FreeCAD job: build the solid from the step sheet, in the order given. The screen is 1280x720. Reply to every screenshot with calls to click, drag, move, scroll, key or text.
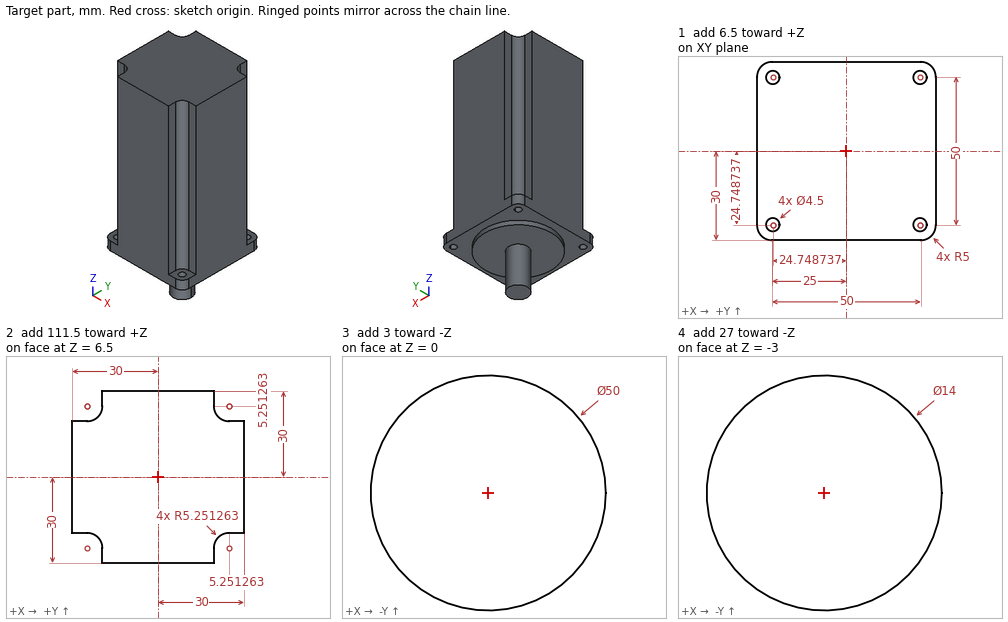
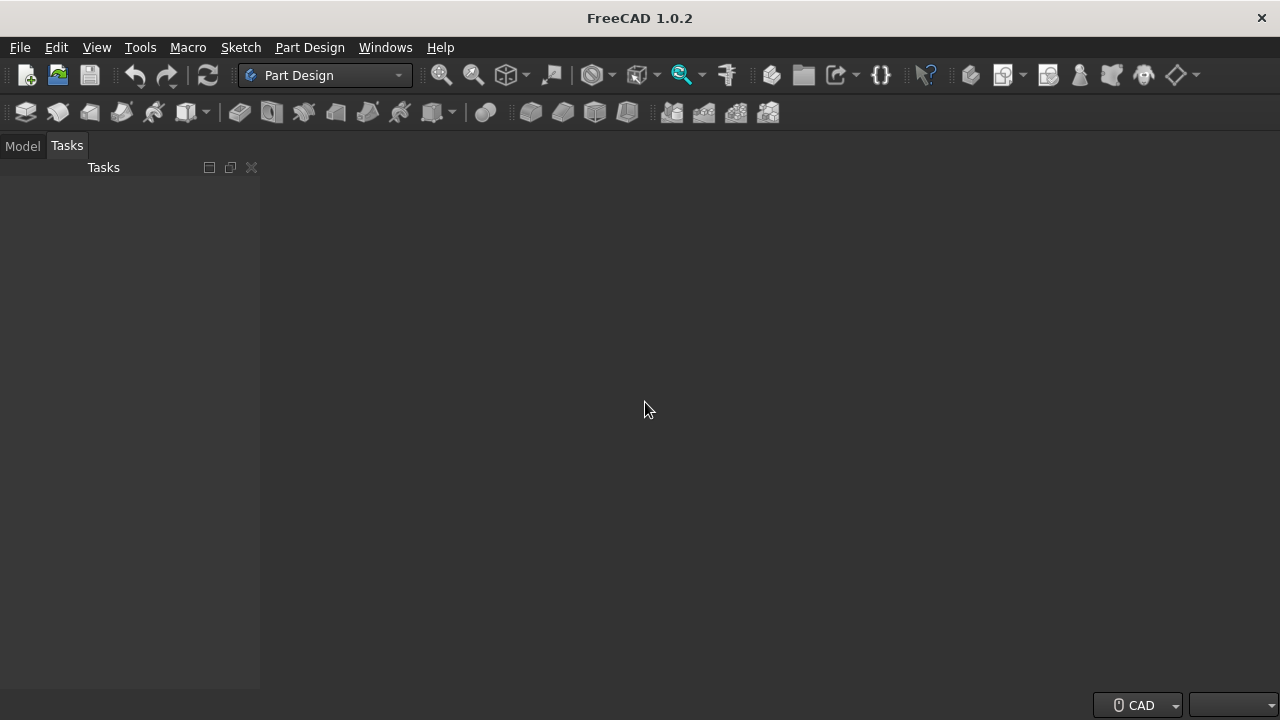
key(ctrl+n)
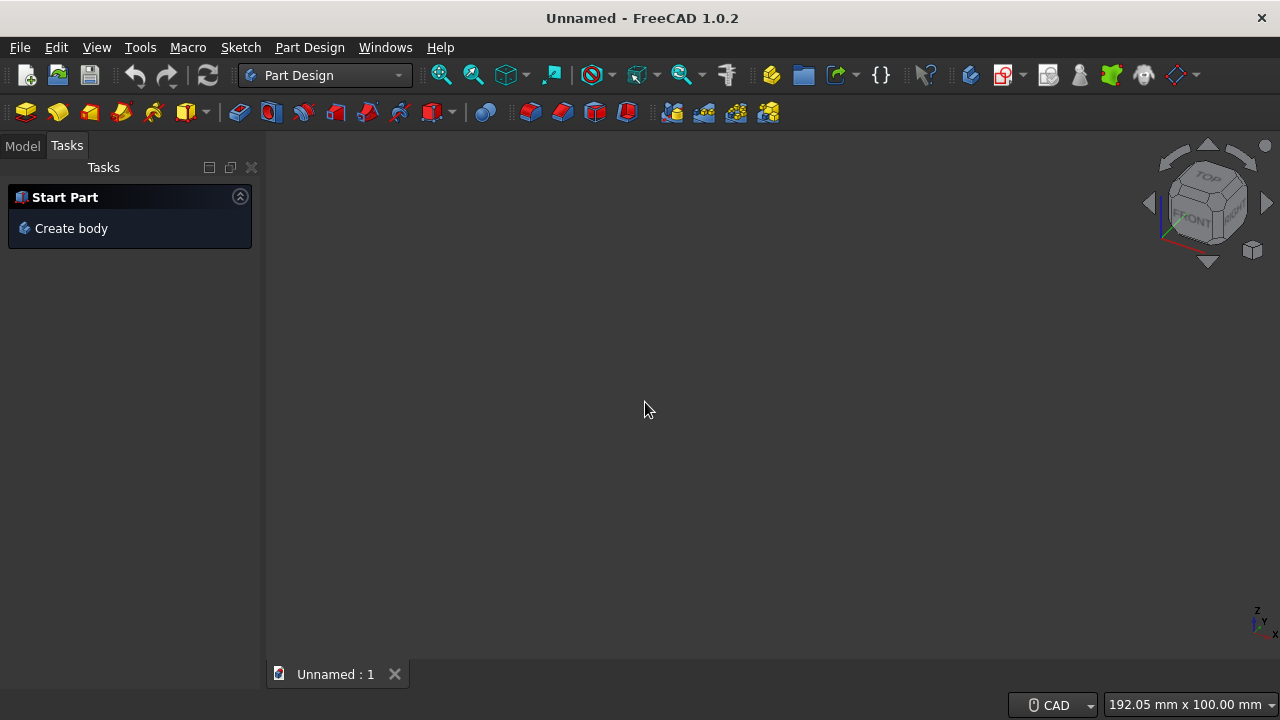
click(1004, 76)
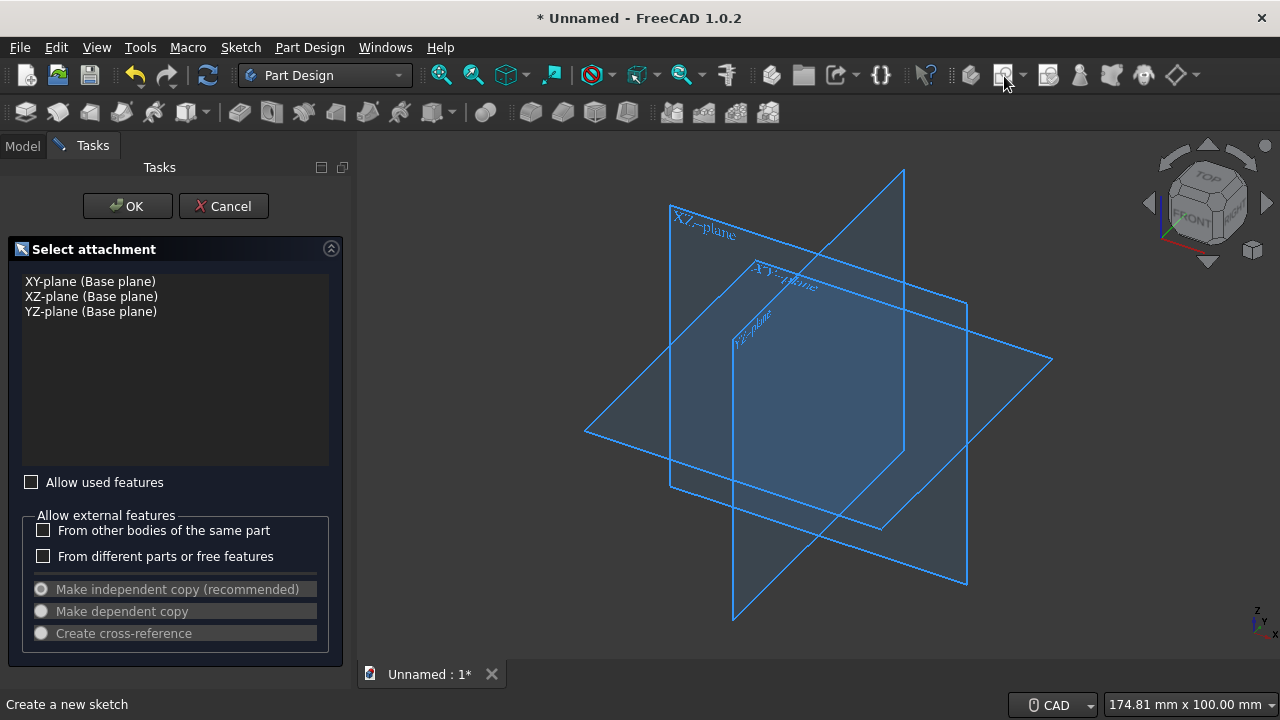
click(82, 282)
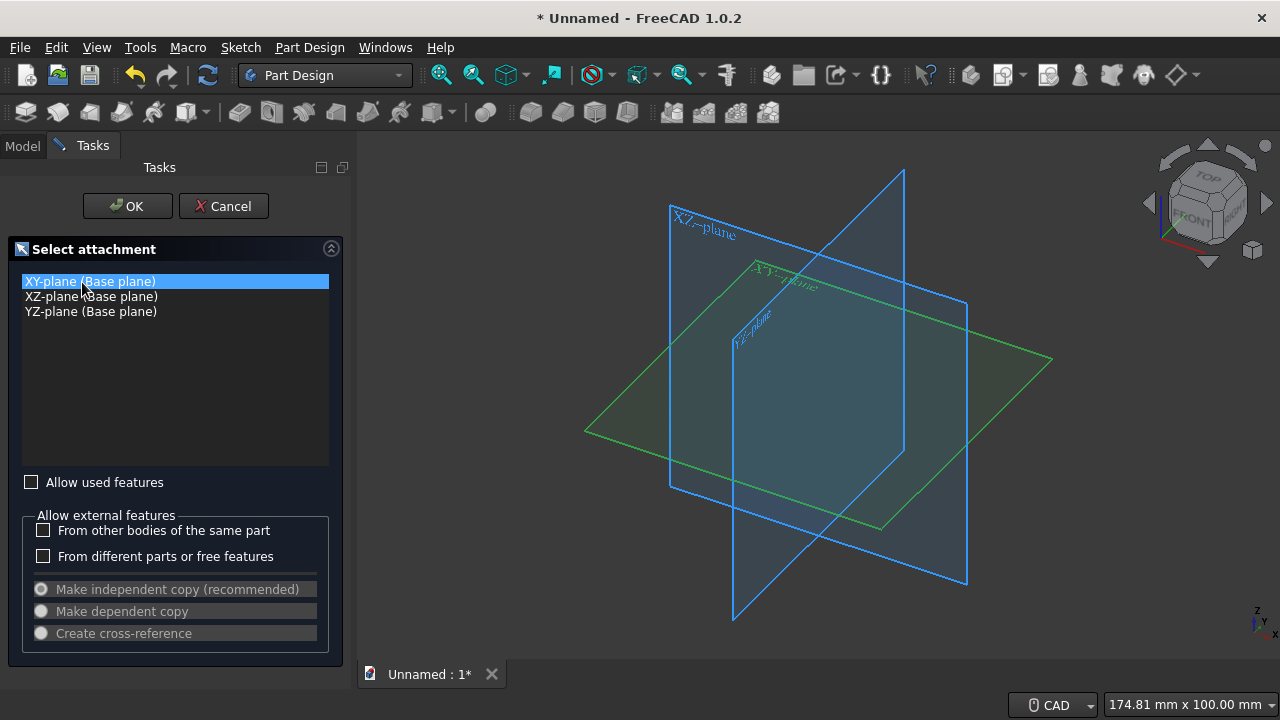
click(128, 206)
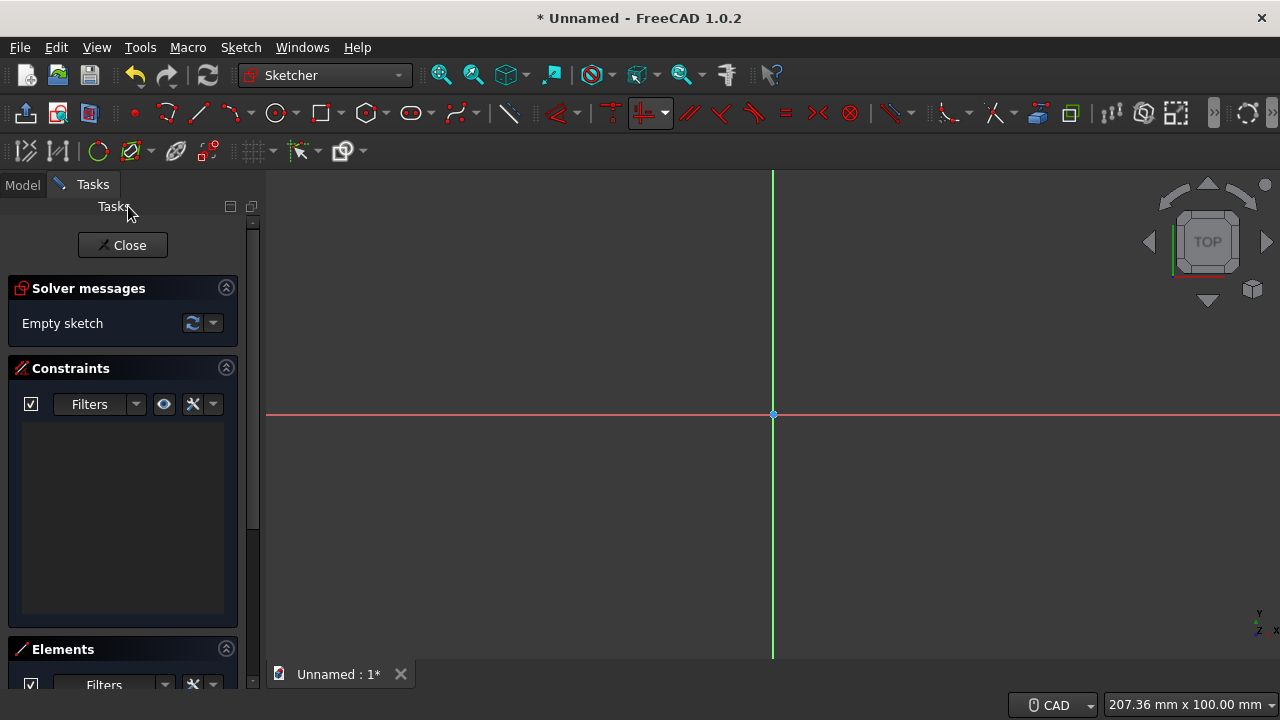
key(g)
key(l)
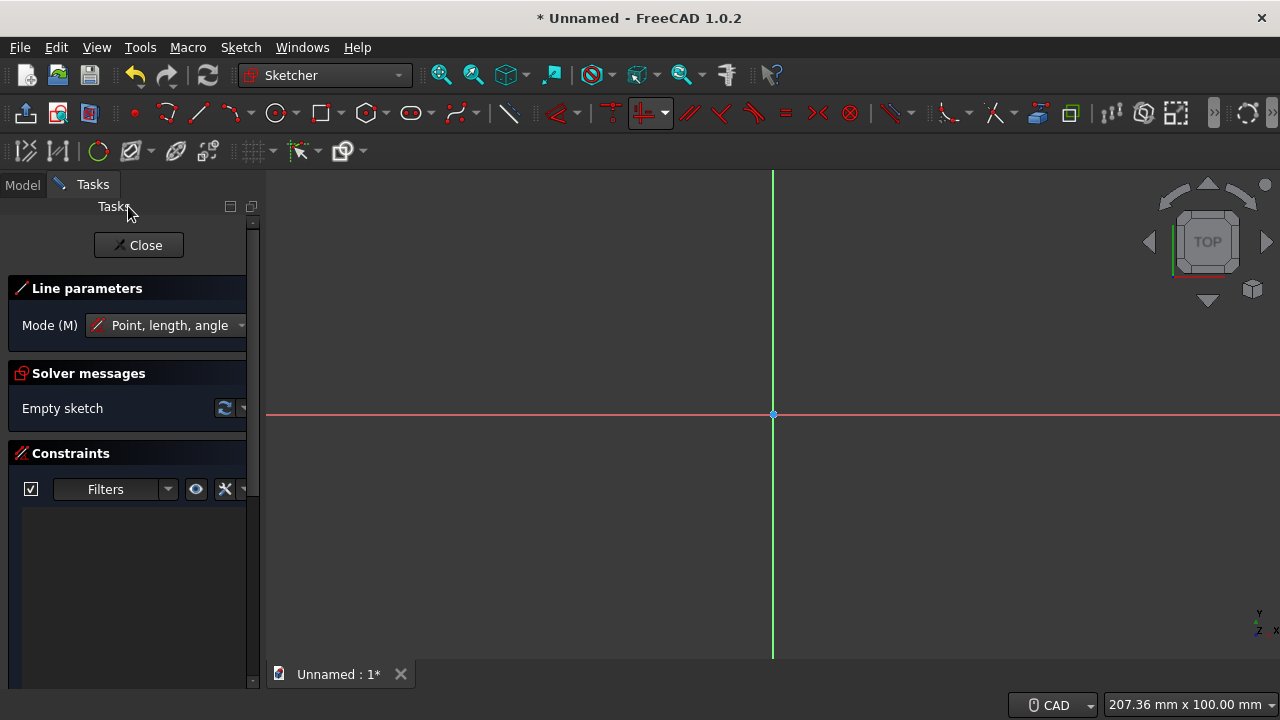
click(651, 561)
click(895, 561)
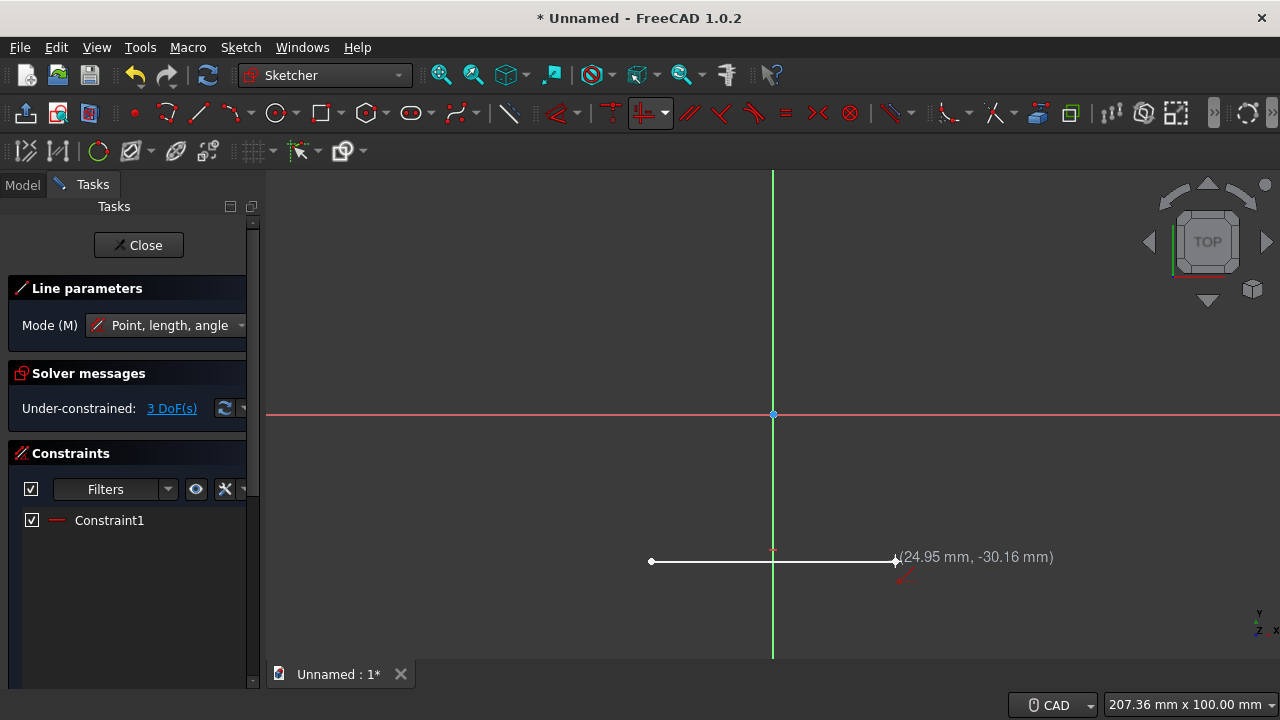
click(920, 537)
click(920, 292)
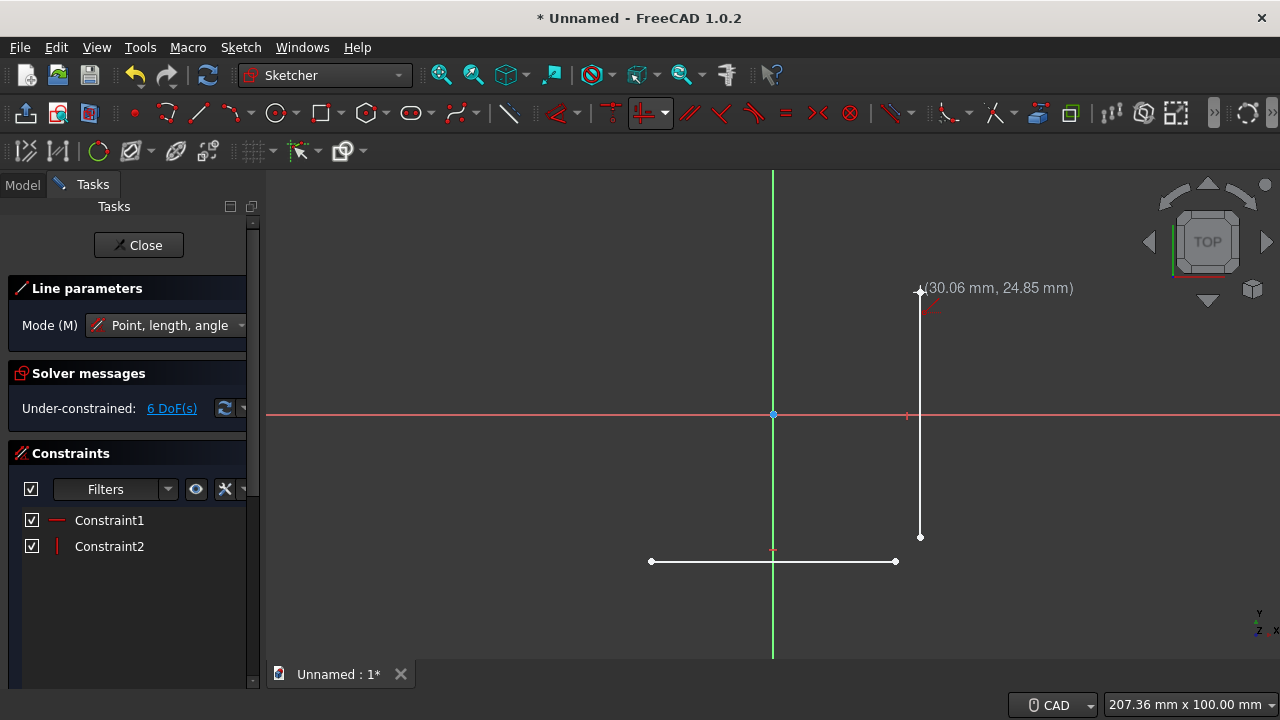
click(895, 268)
click(651, 268)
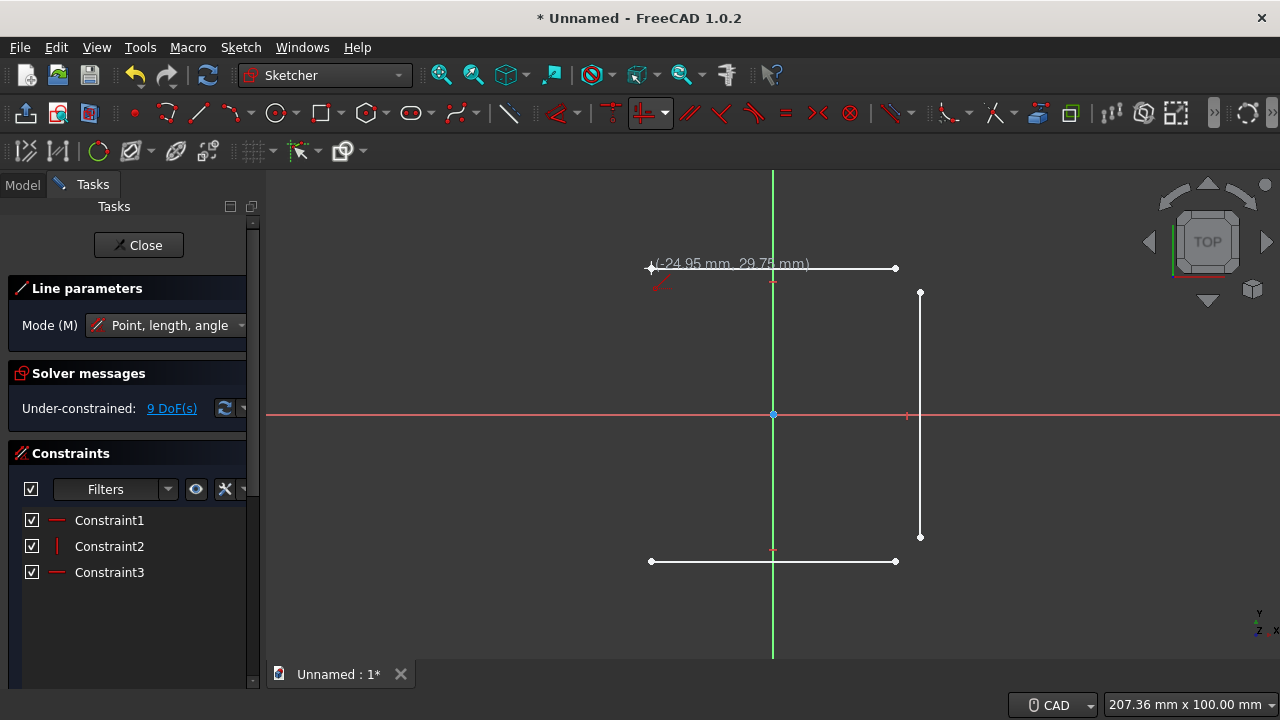
click(626, 292)
click(626, 537)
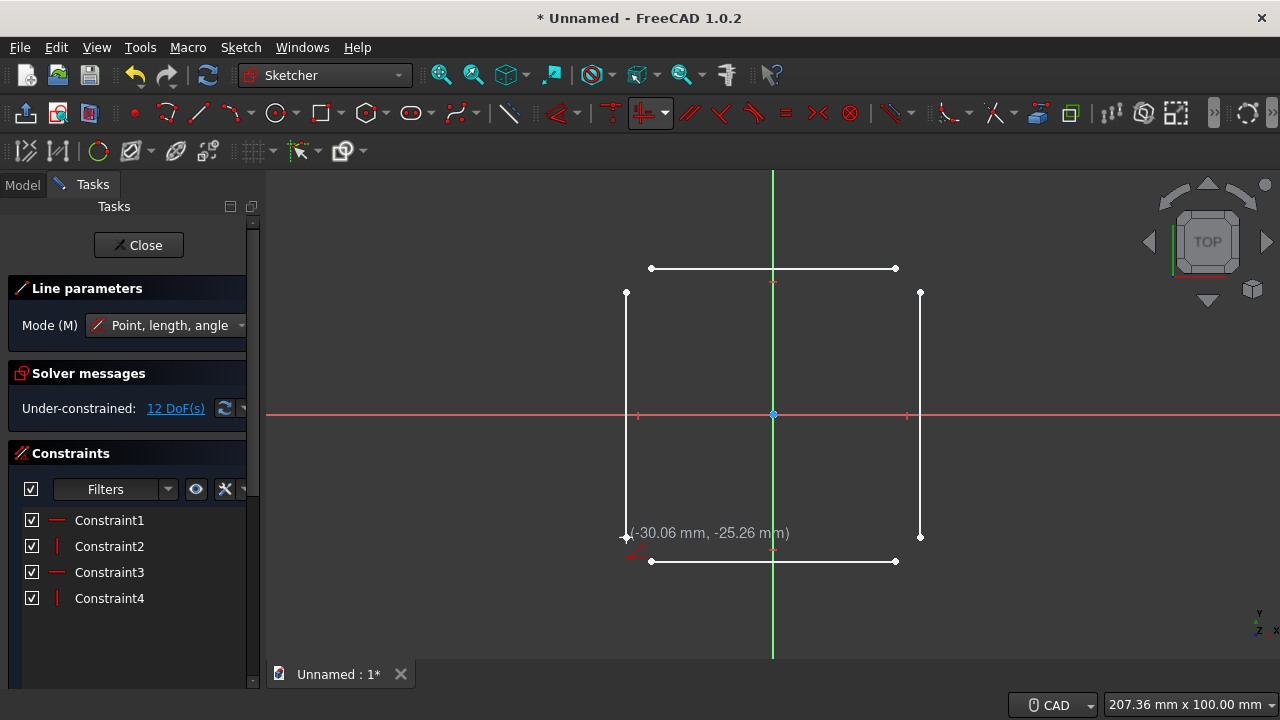
click(232, 114)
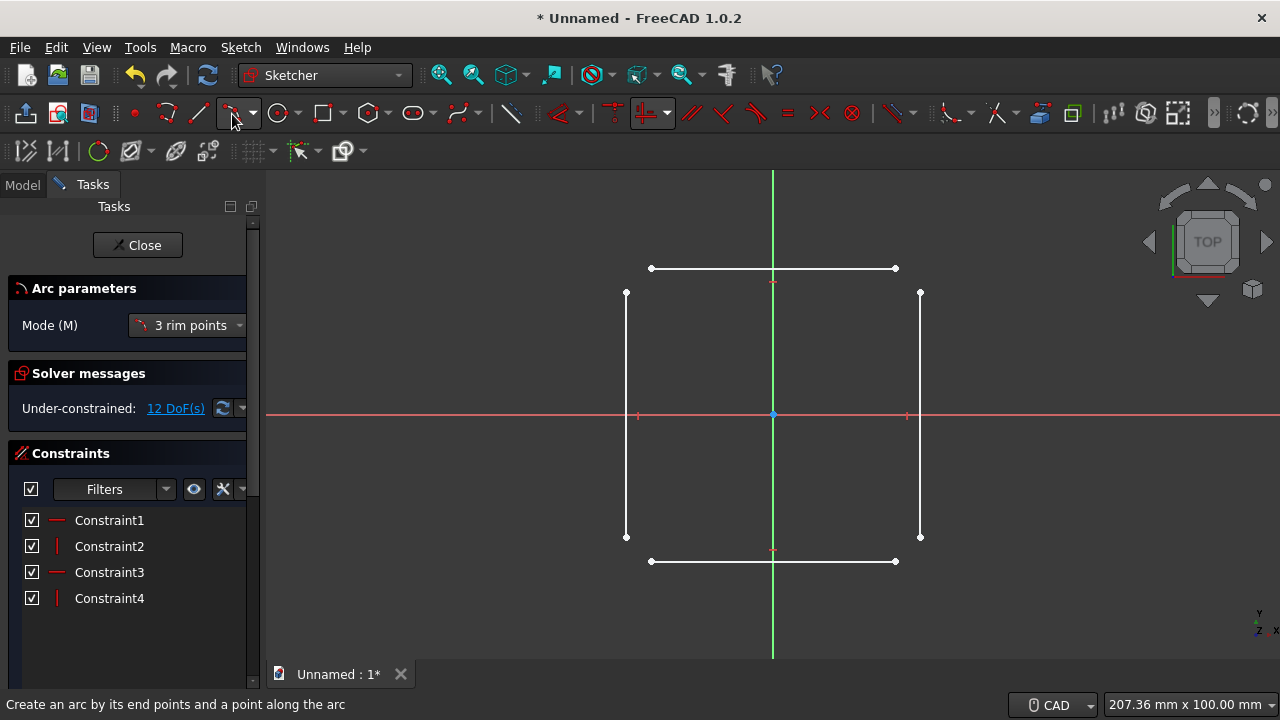
click(895, 562)
click(920, 538)